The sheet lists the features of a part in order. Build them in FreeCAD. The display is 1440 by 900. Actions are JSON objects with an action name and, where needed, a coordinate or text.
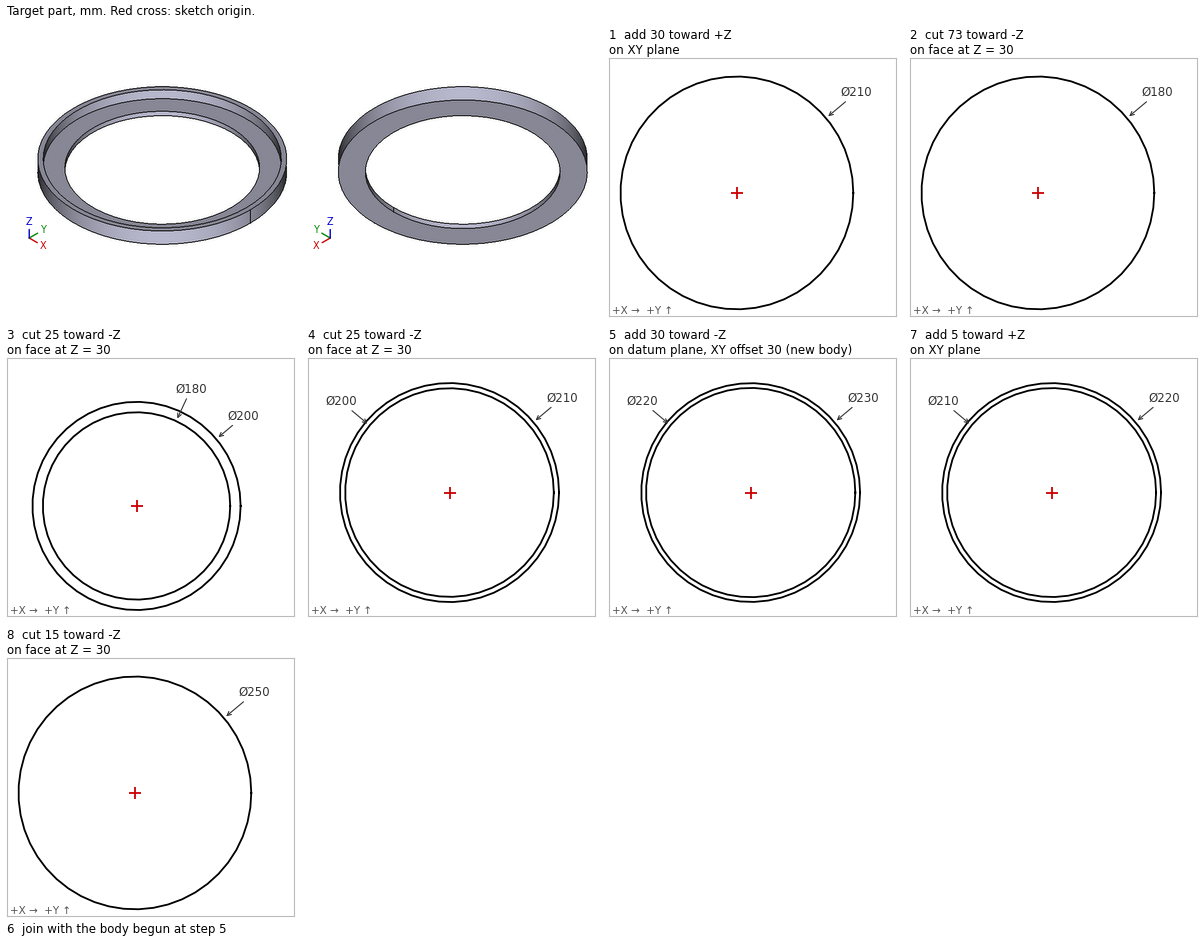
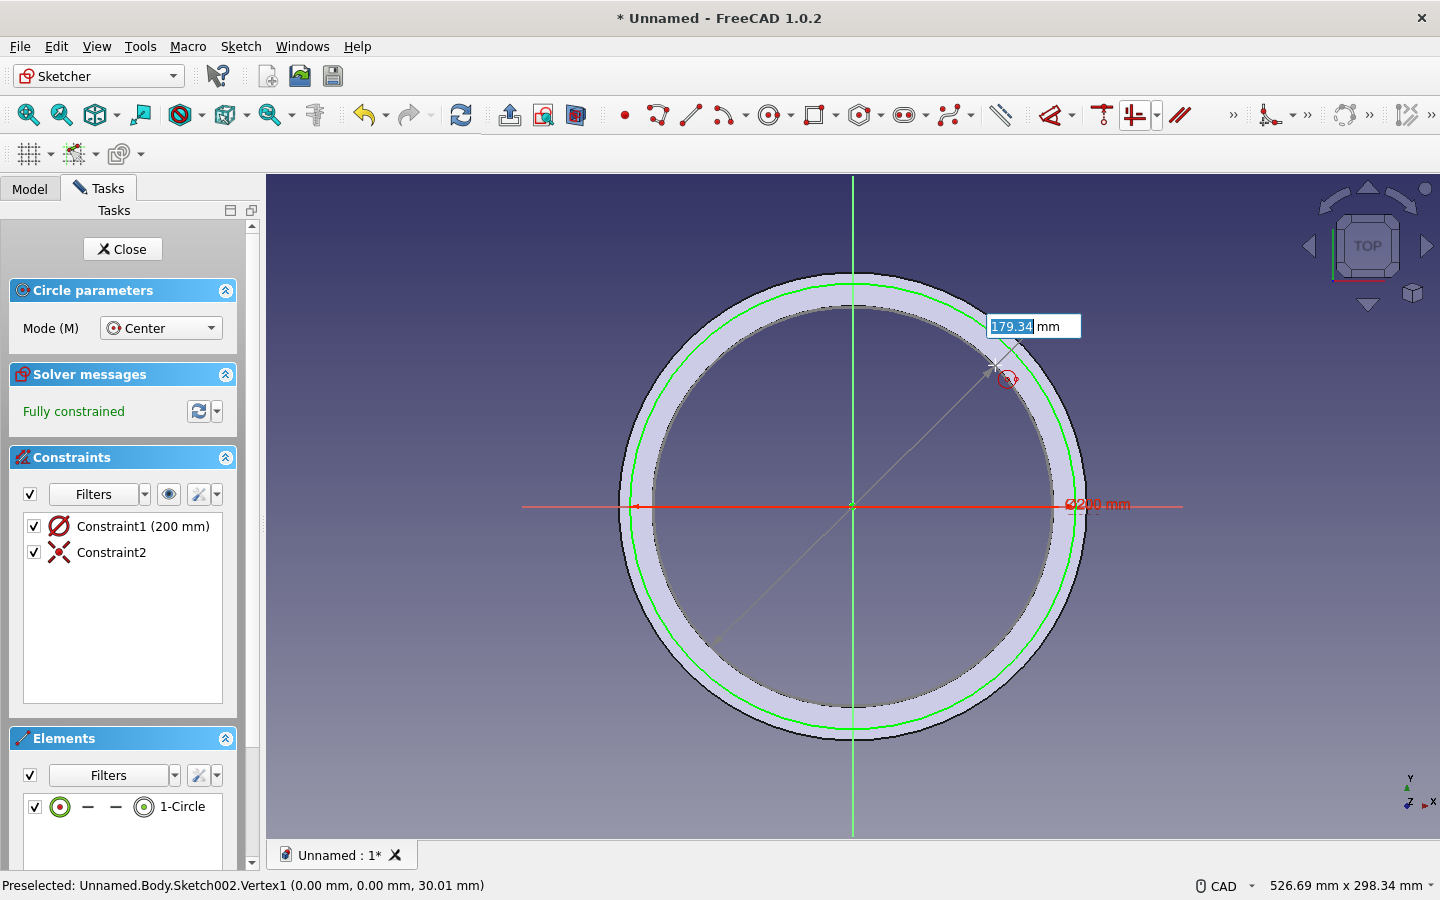
{"action": "type", "text": "180"}
{"action": "key", "text": "Return"}
{"action": "key", "text": "Escape"}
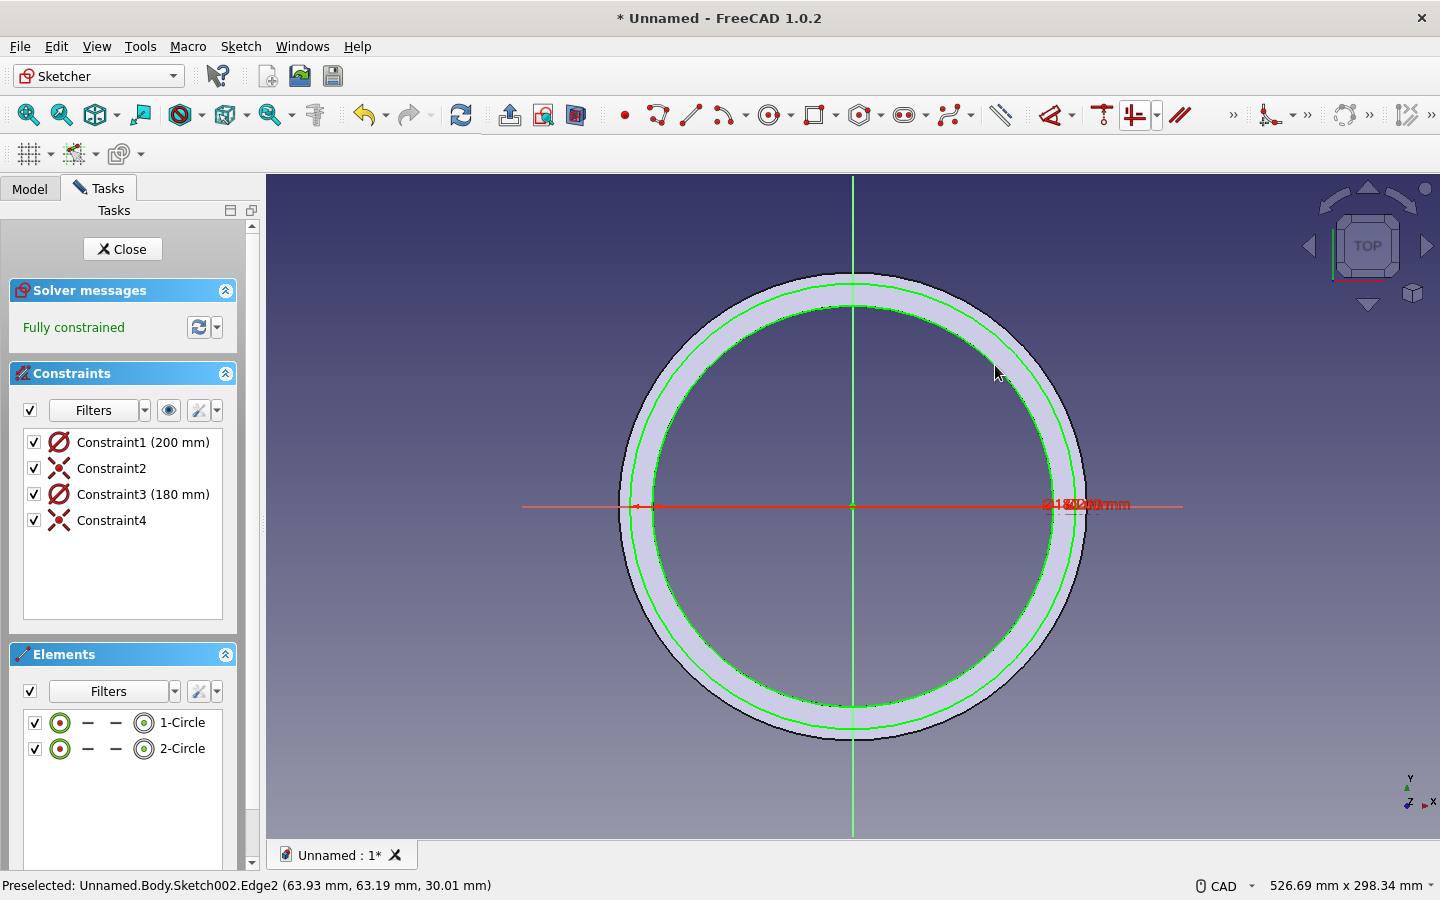
{"action": "left_click", "coordinate": [123, 249]}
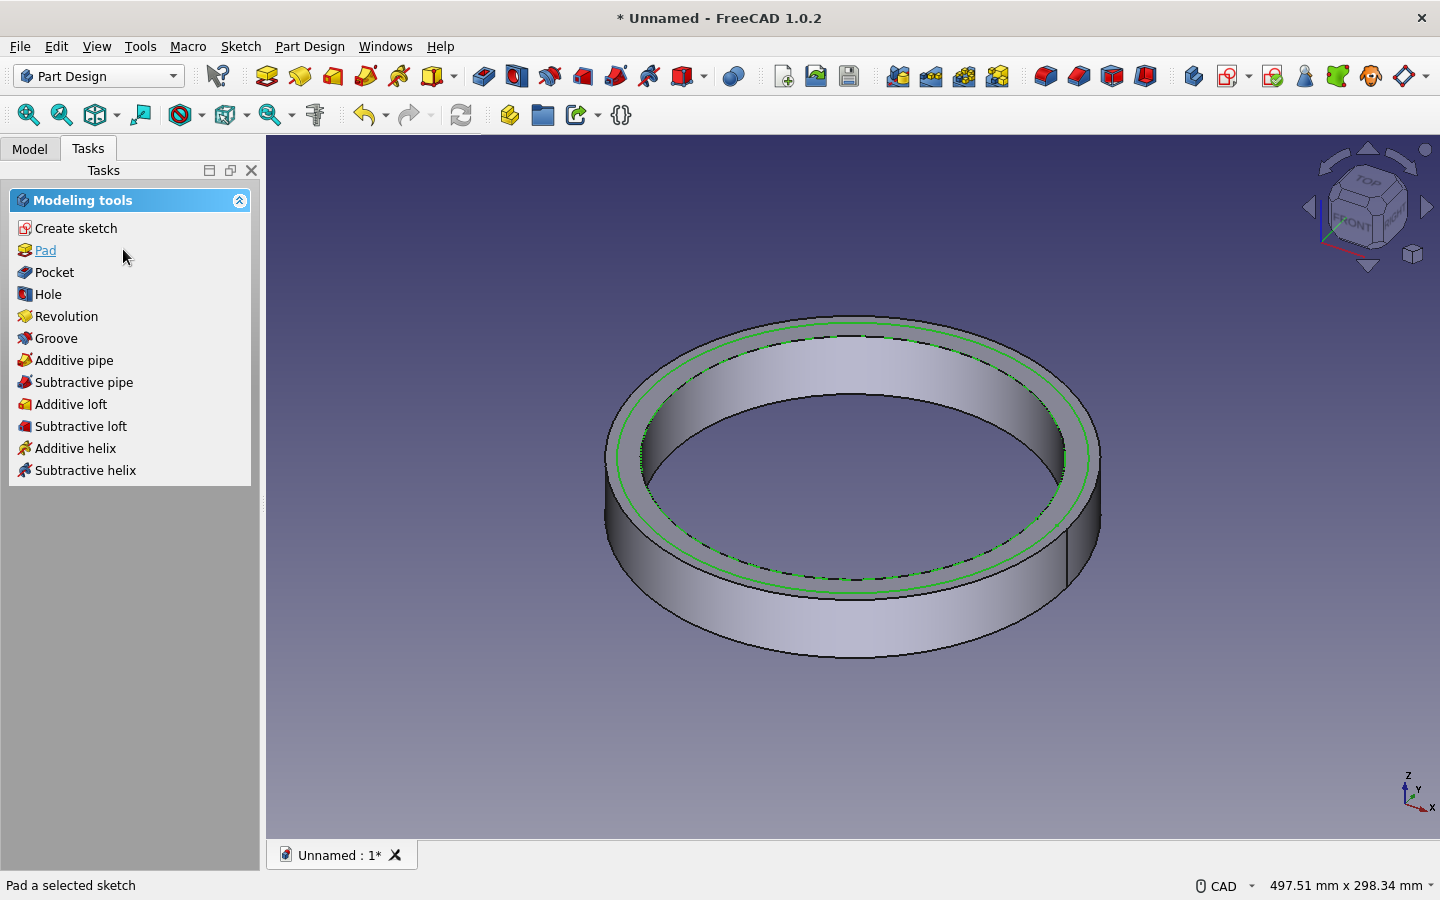
{"action": "left_click", "coordinate": [484, 76]}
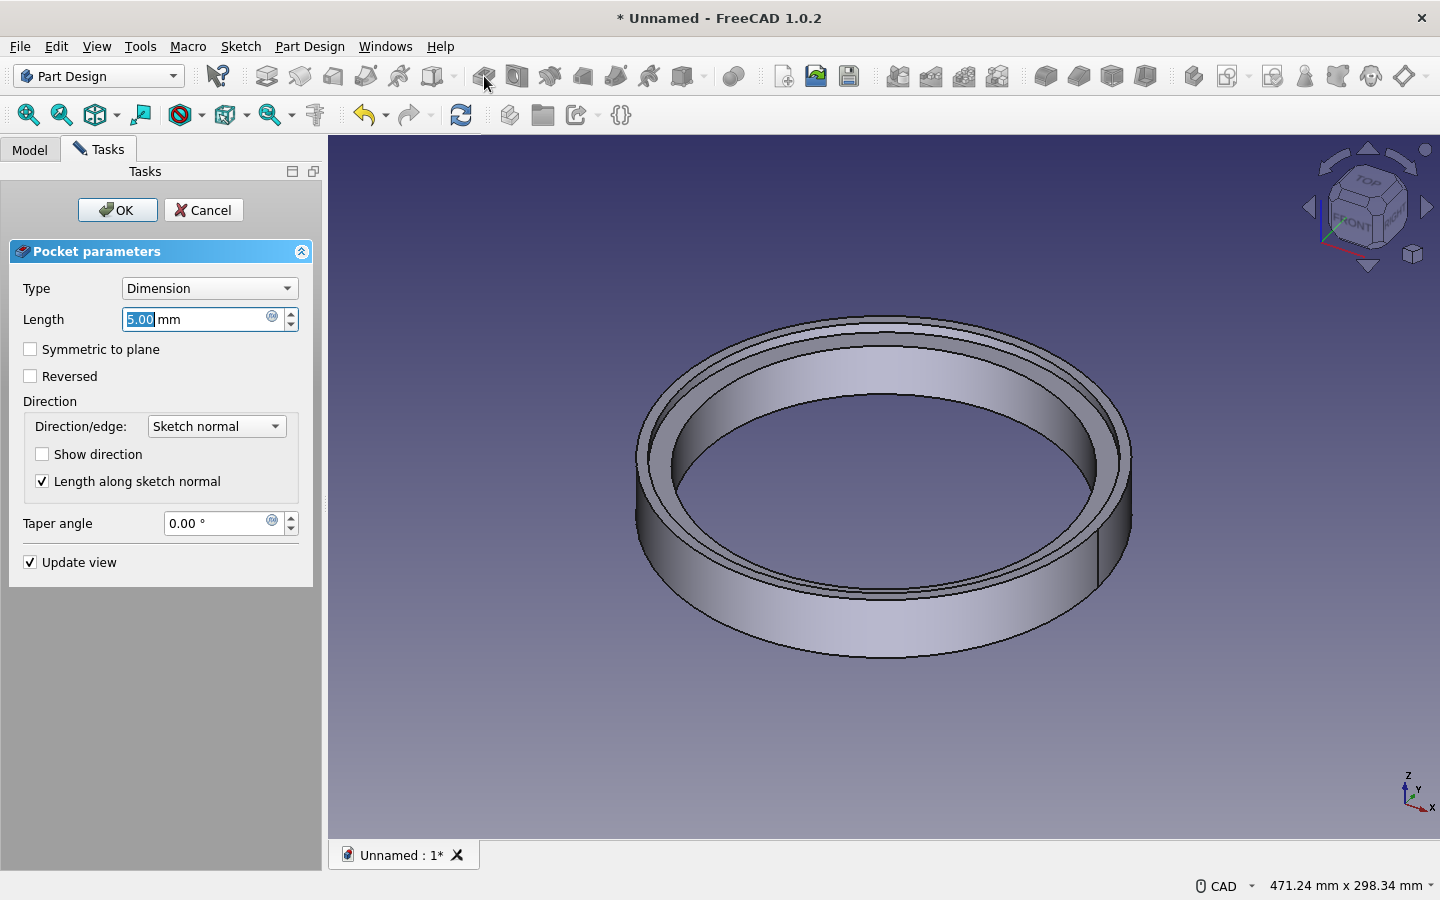
{"action": "type", "text": "25"}
{"action": "key", "text": "Tab"}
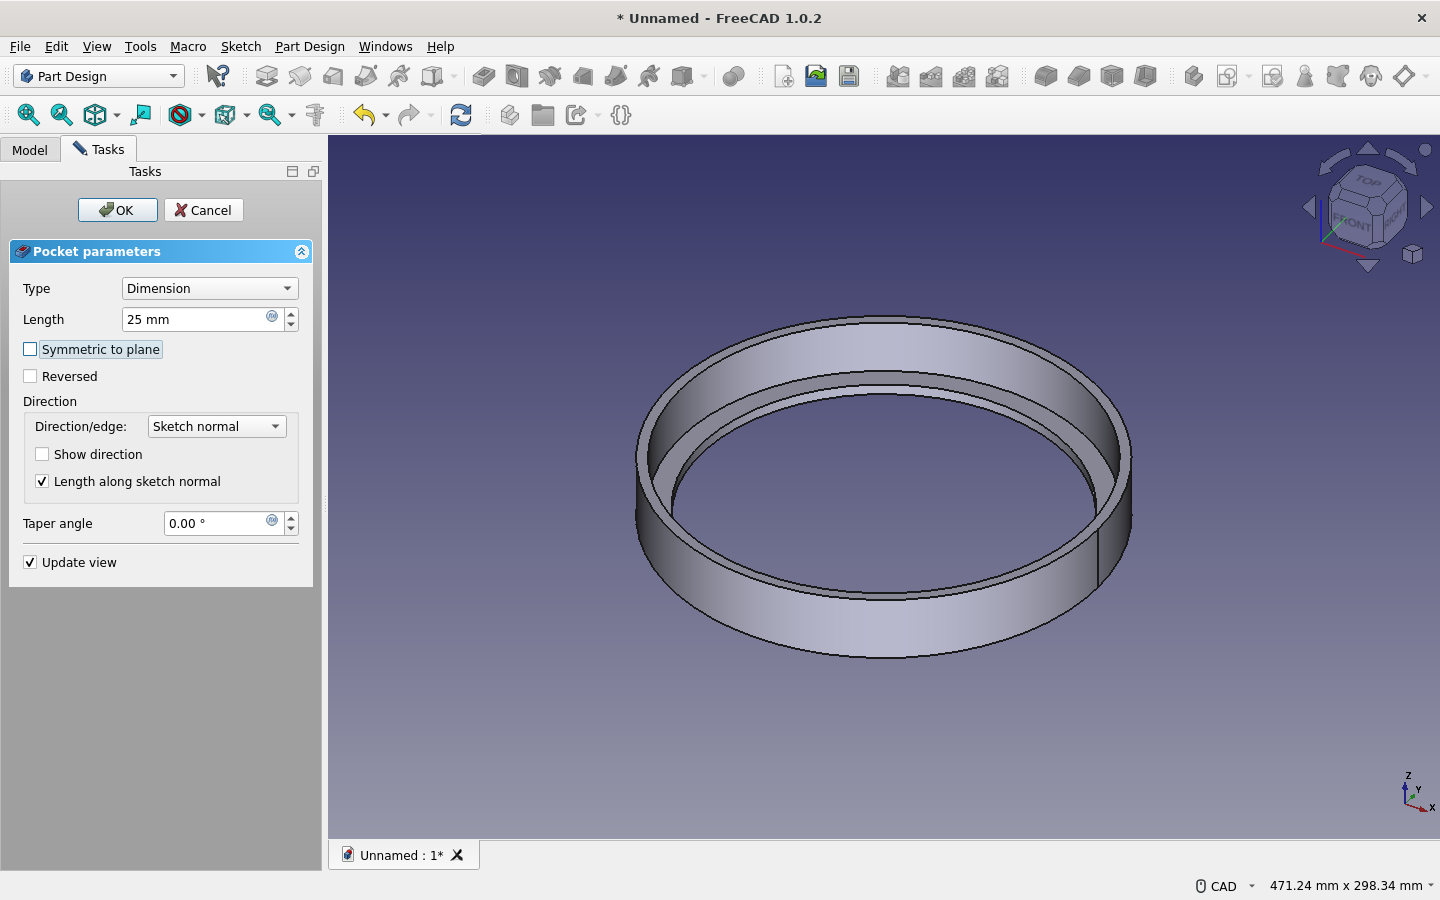
{"action": "left_click", "coordinate": [118, 210]}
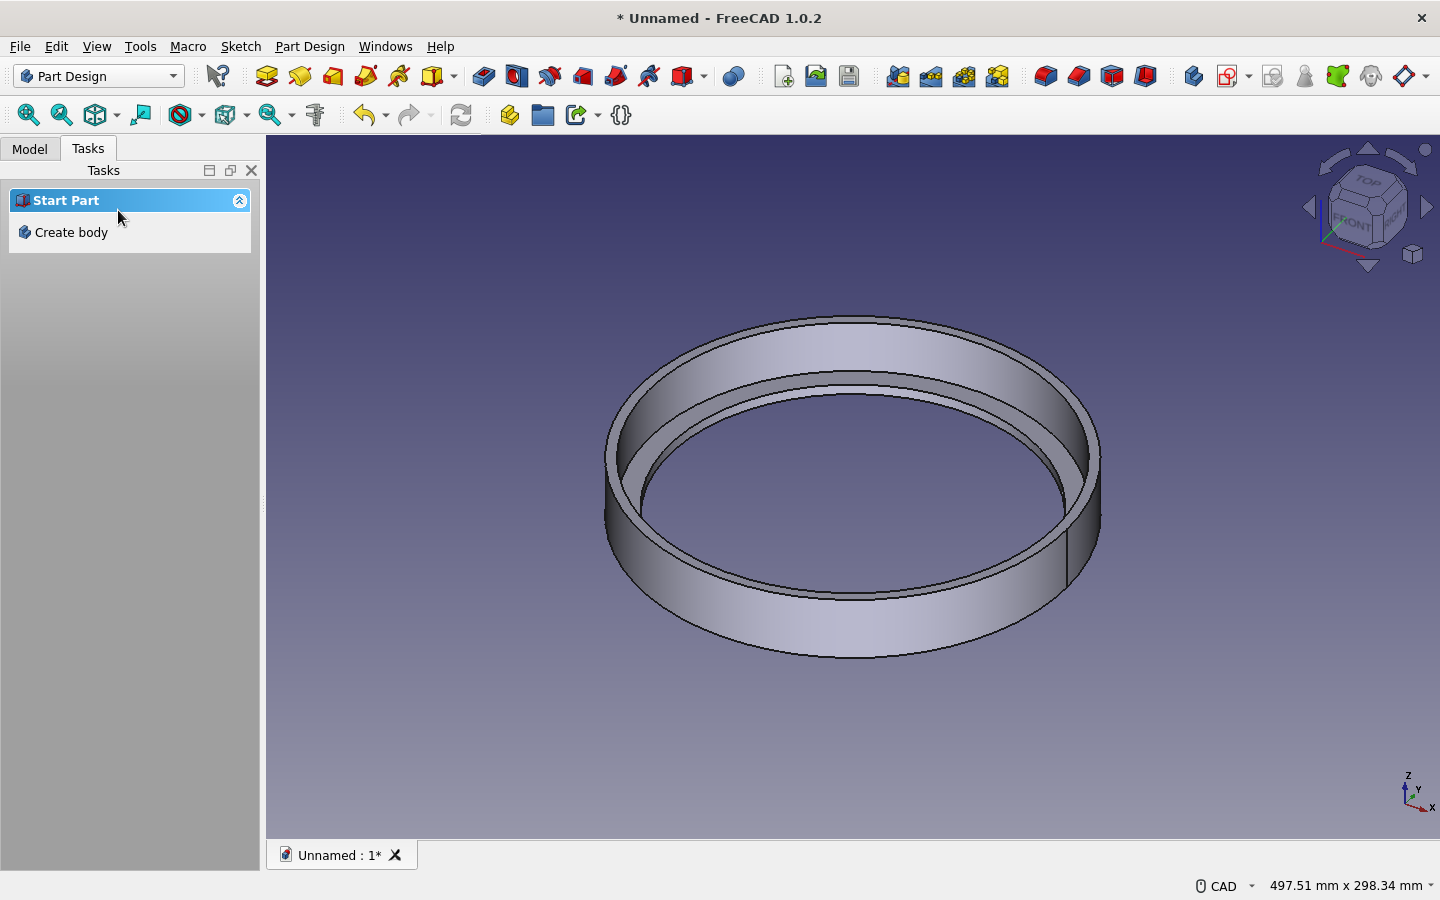
{"action": "scroll", "coordinate": [789, 592], "scroll_direction": "up", "scroll_amount": 6}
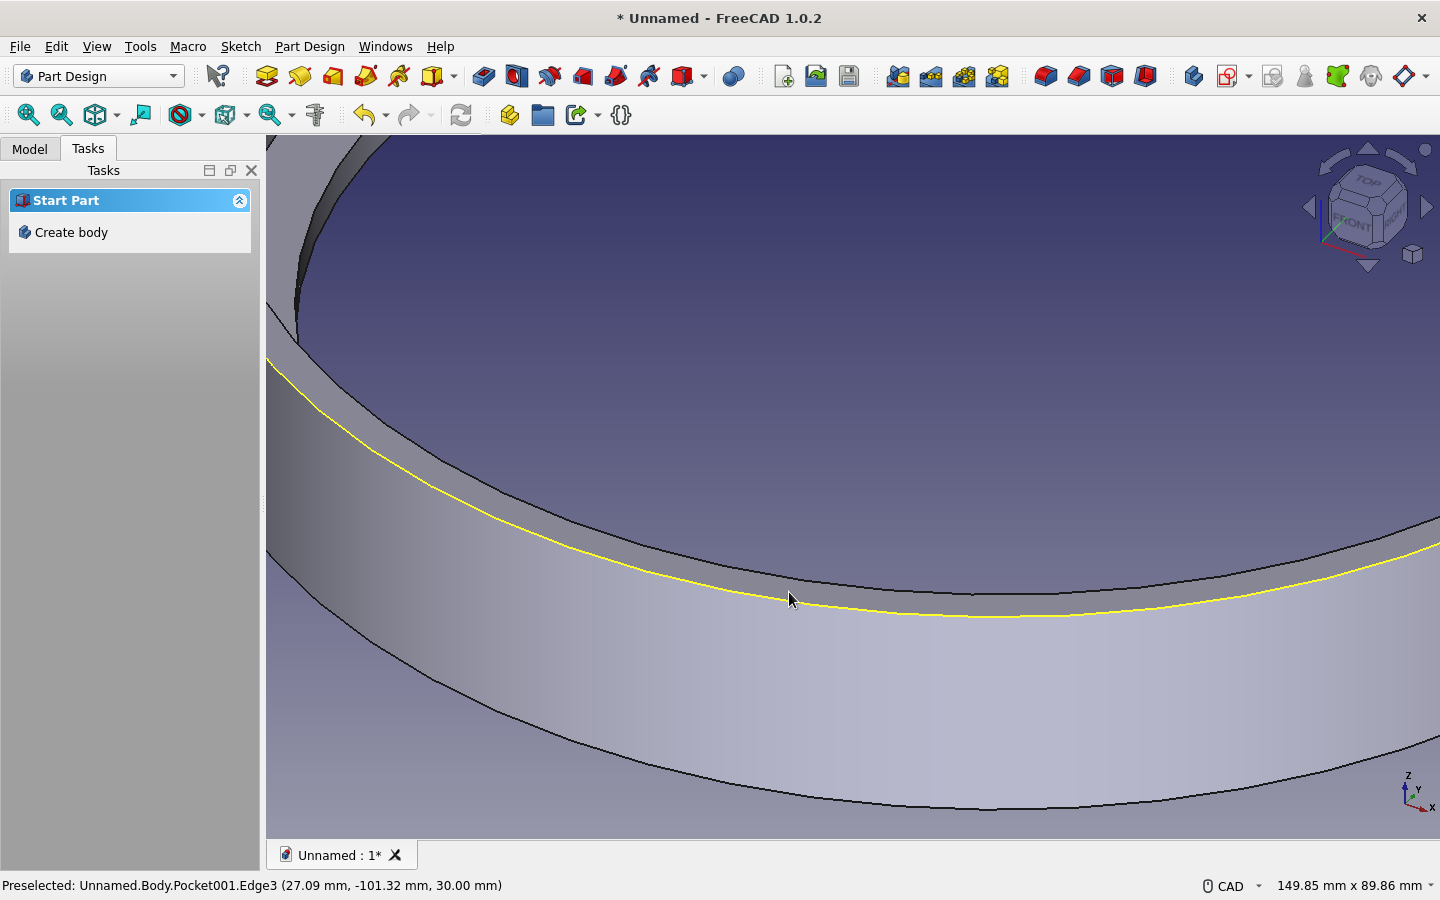
{"action": "left_click", "coordinate": [29, 116]}